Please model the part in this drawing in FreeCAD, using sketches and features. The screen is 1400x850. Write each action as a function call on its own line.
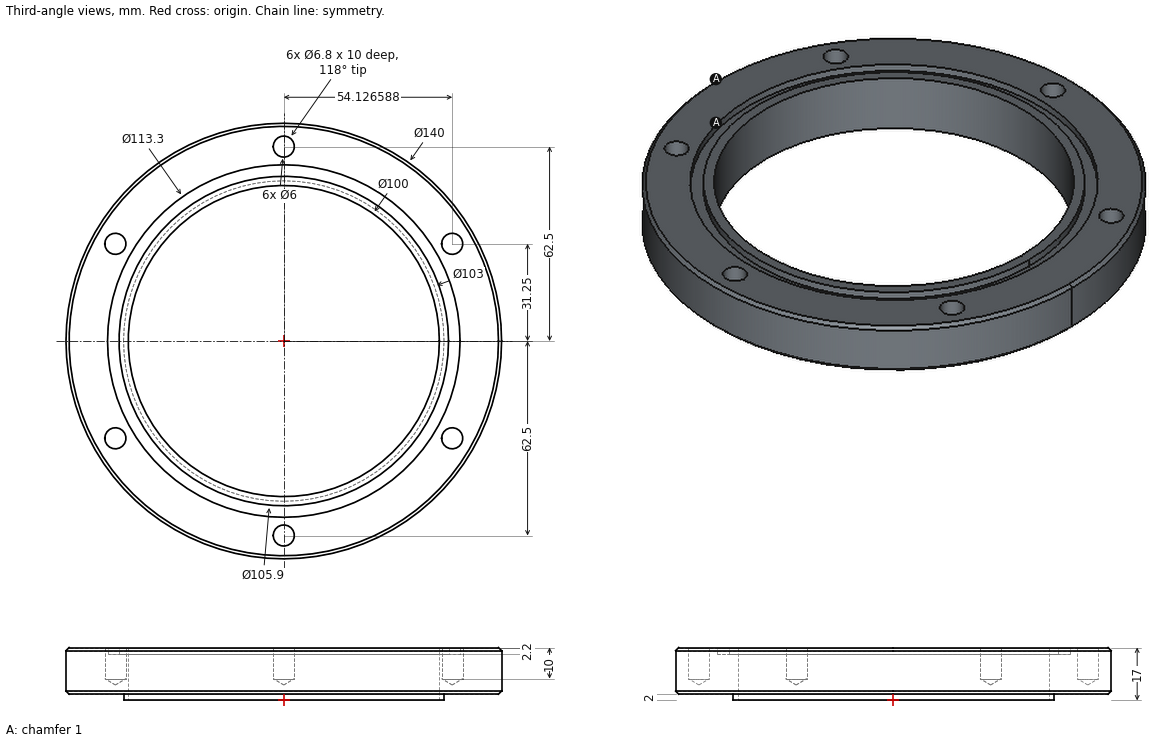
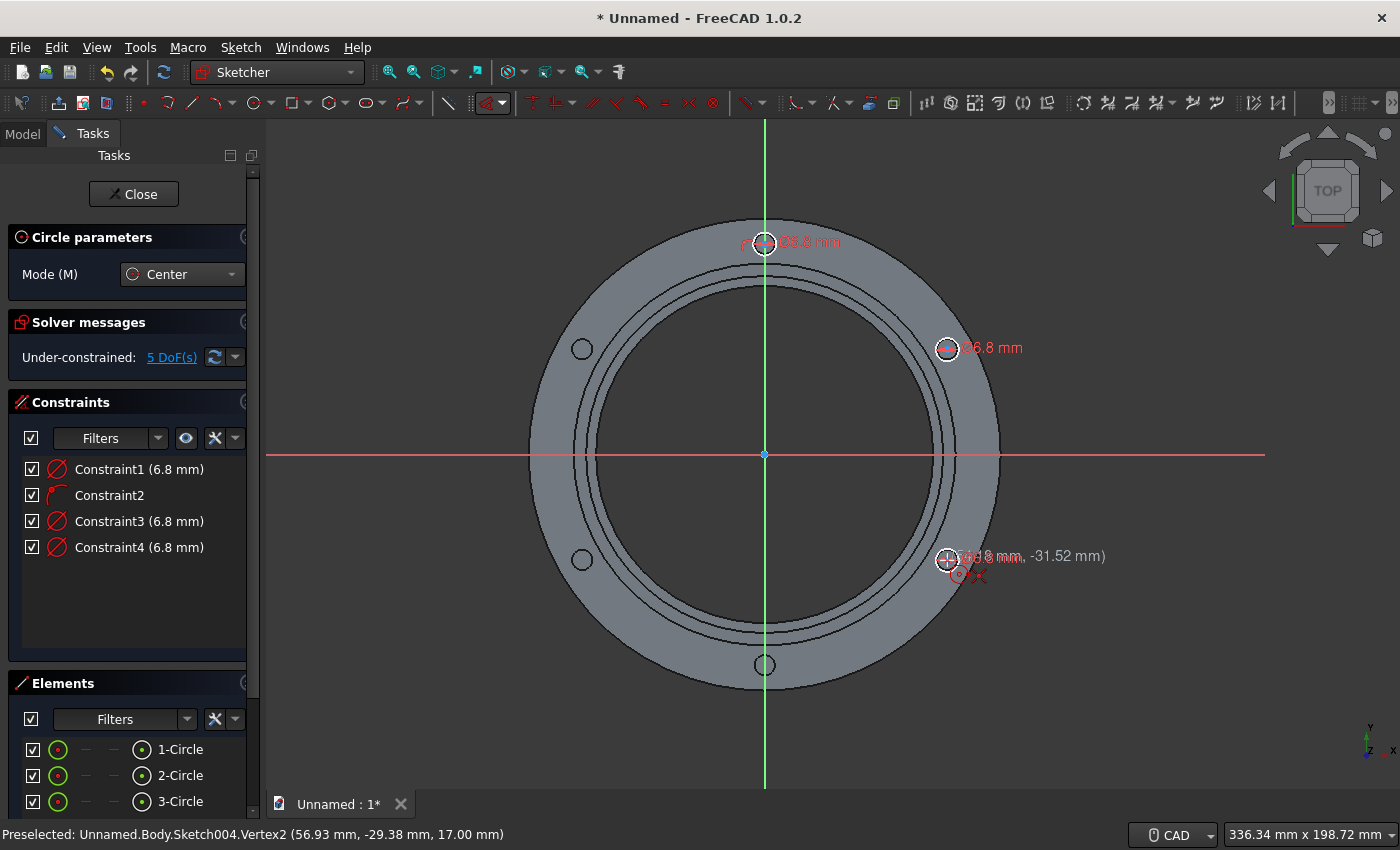
scroll(765, 665, up, 4)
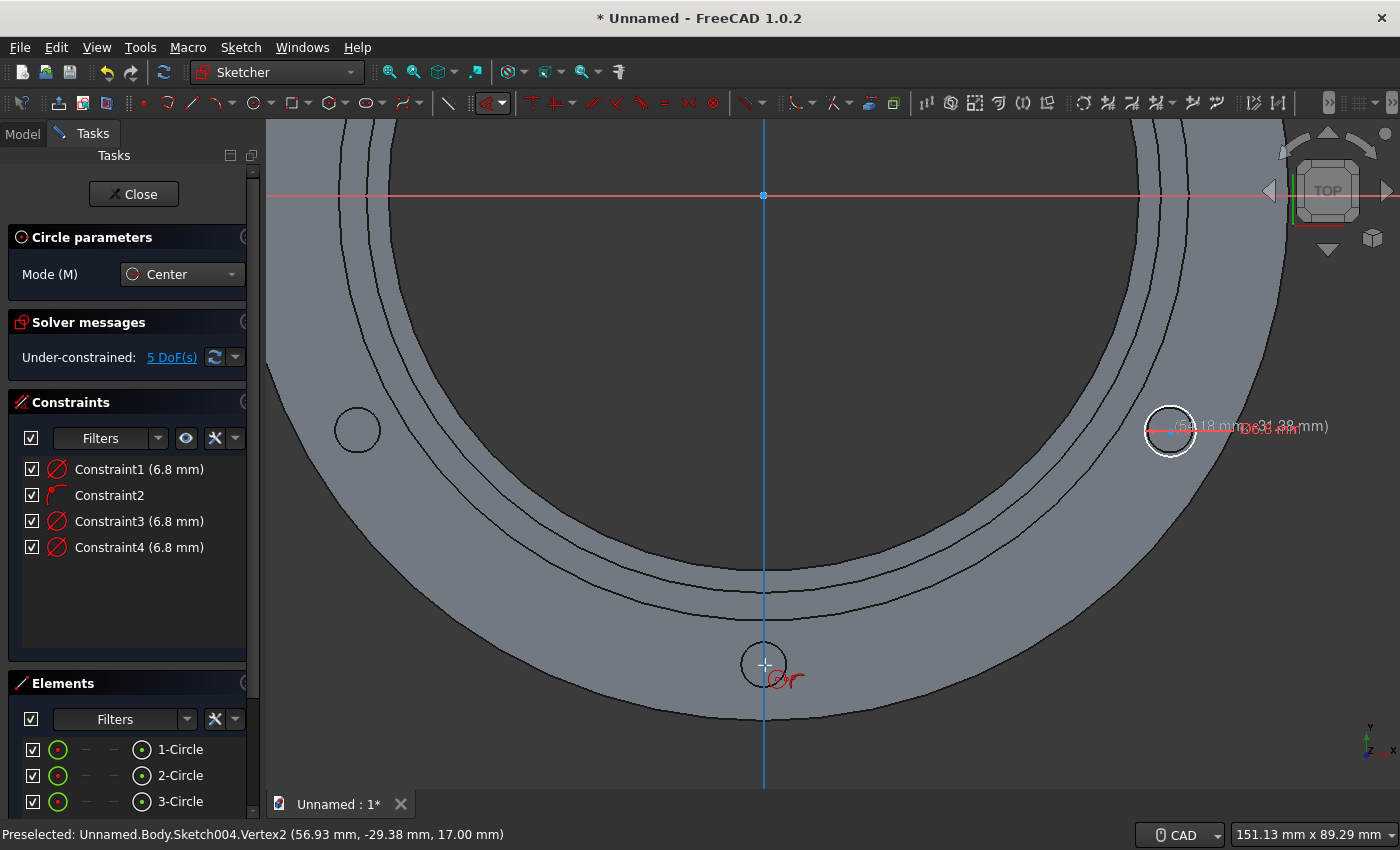
click(764, 665)
move(782, 647)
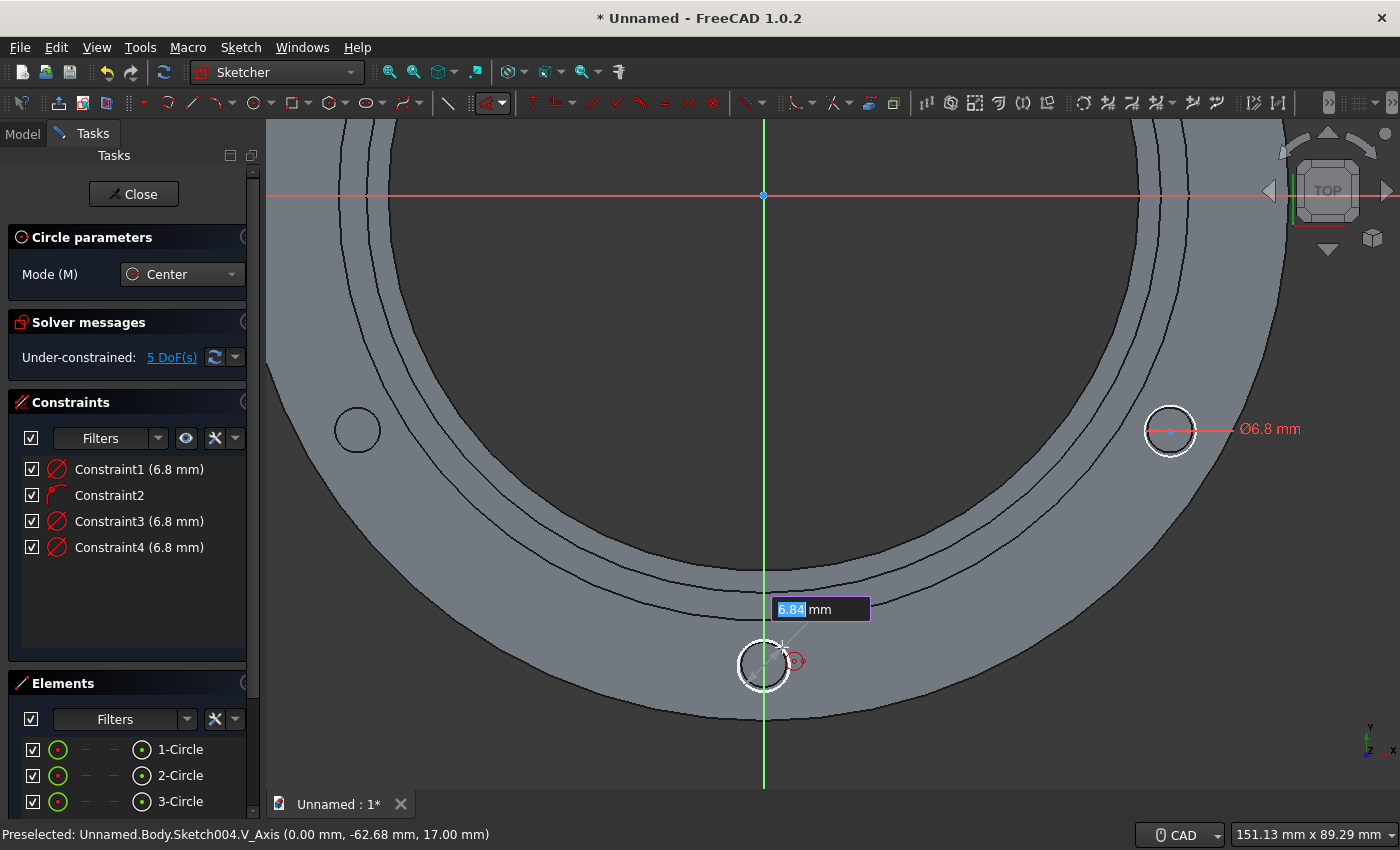
text(6.8)
key(Return)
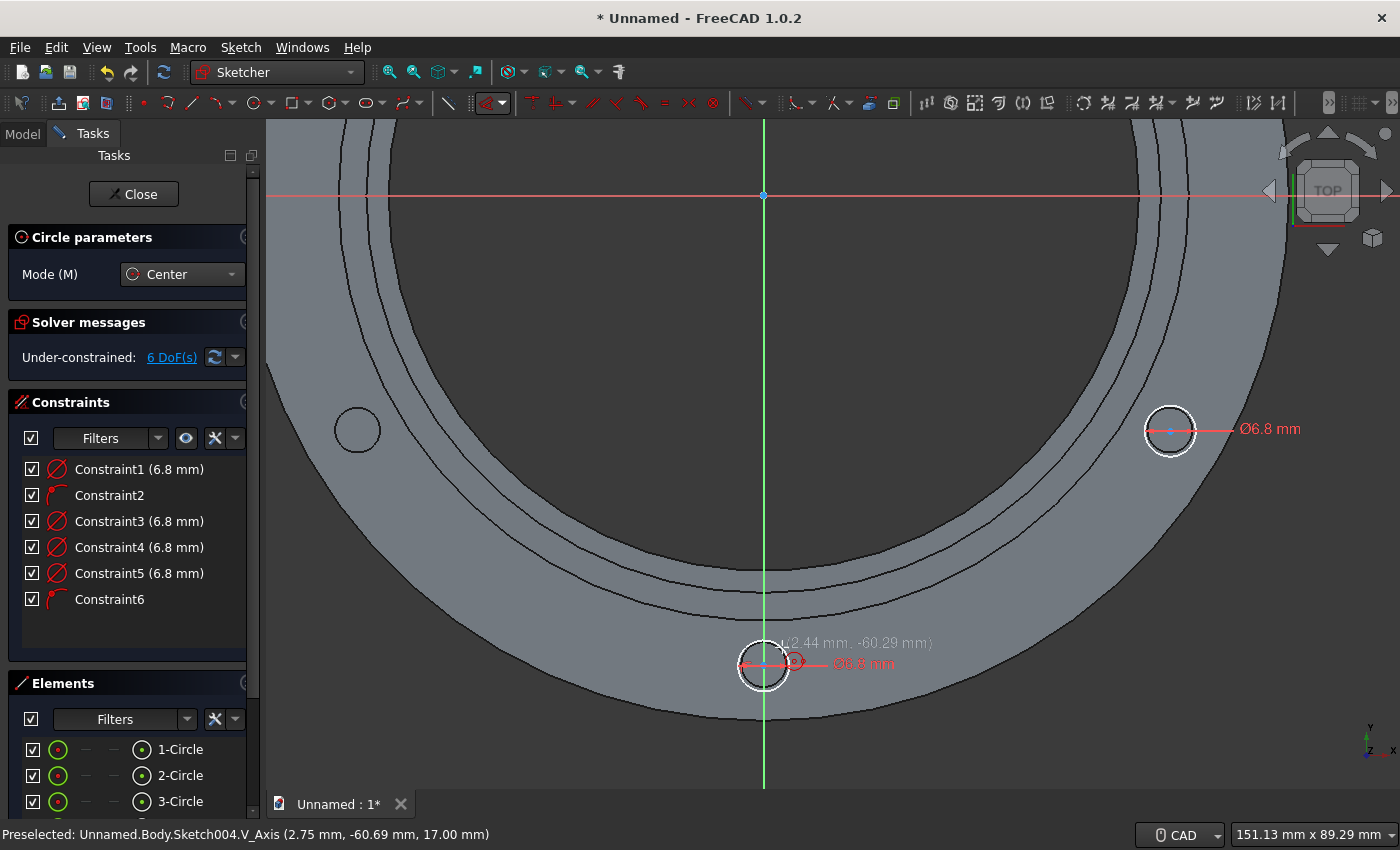
click(358, 430)
move(376, 412)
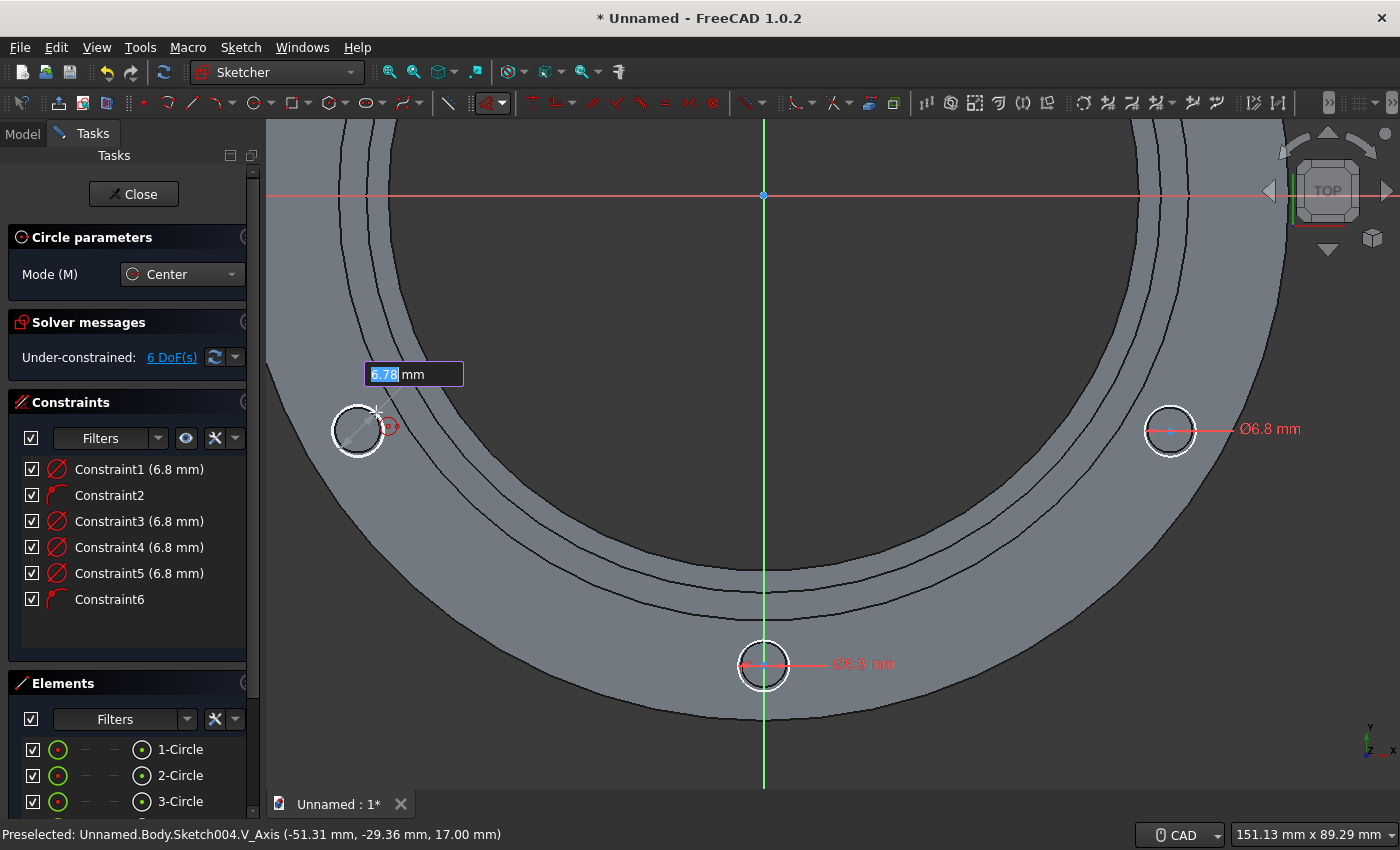
text(6.8)
key(Return)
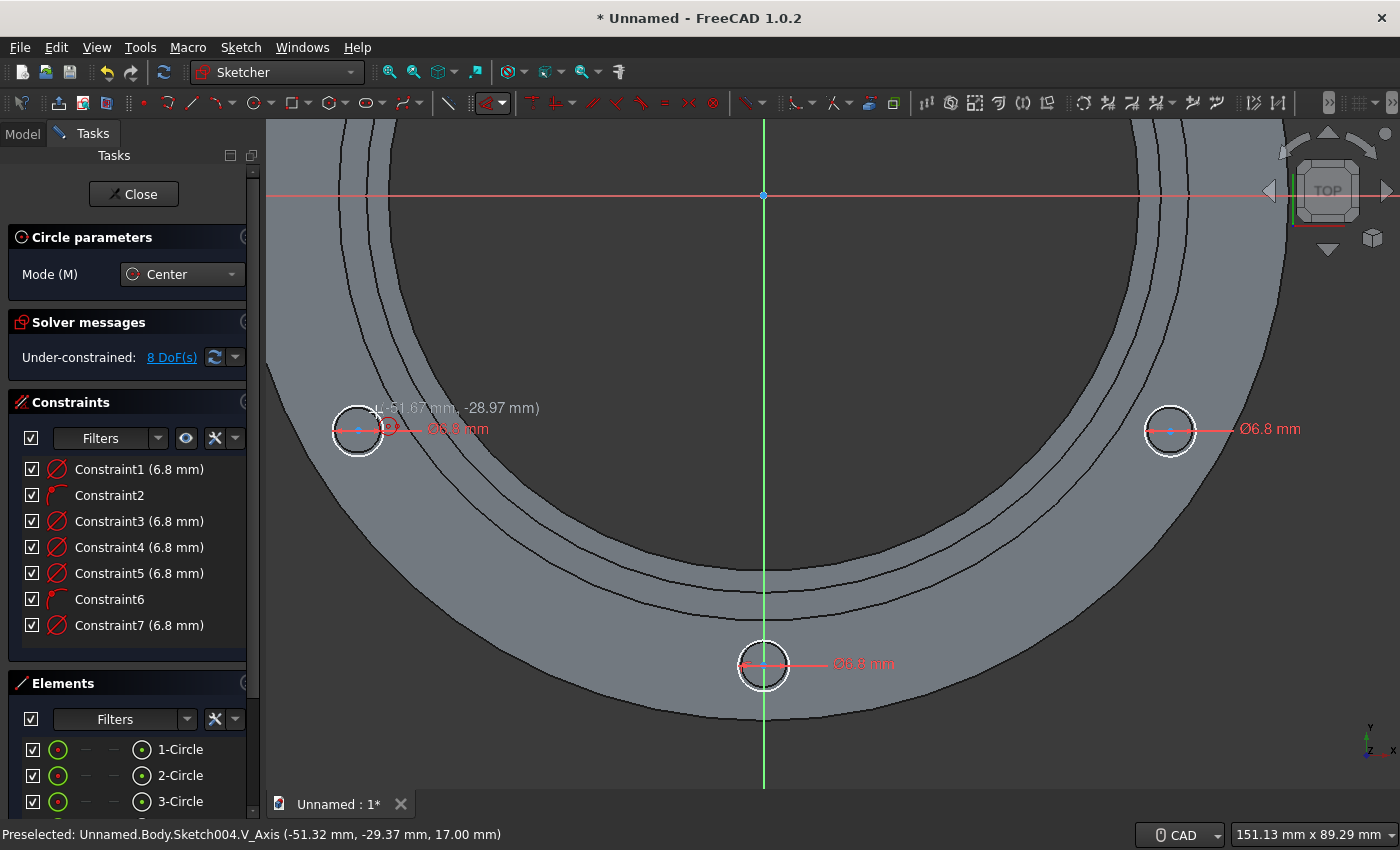
scroll(765, 665, down, 4)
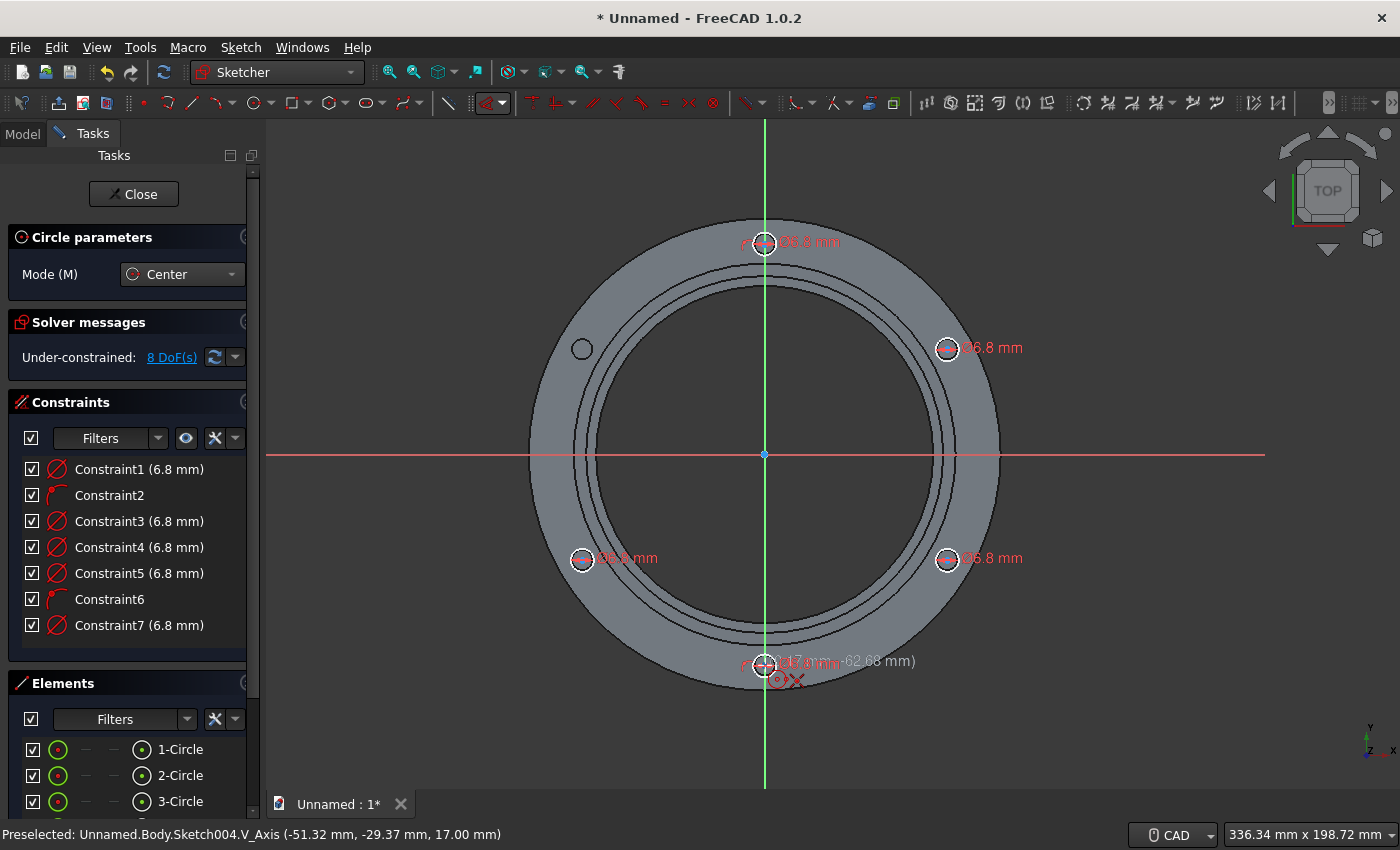
scroll(582, 349, up, 4)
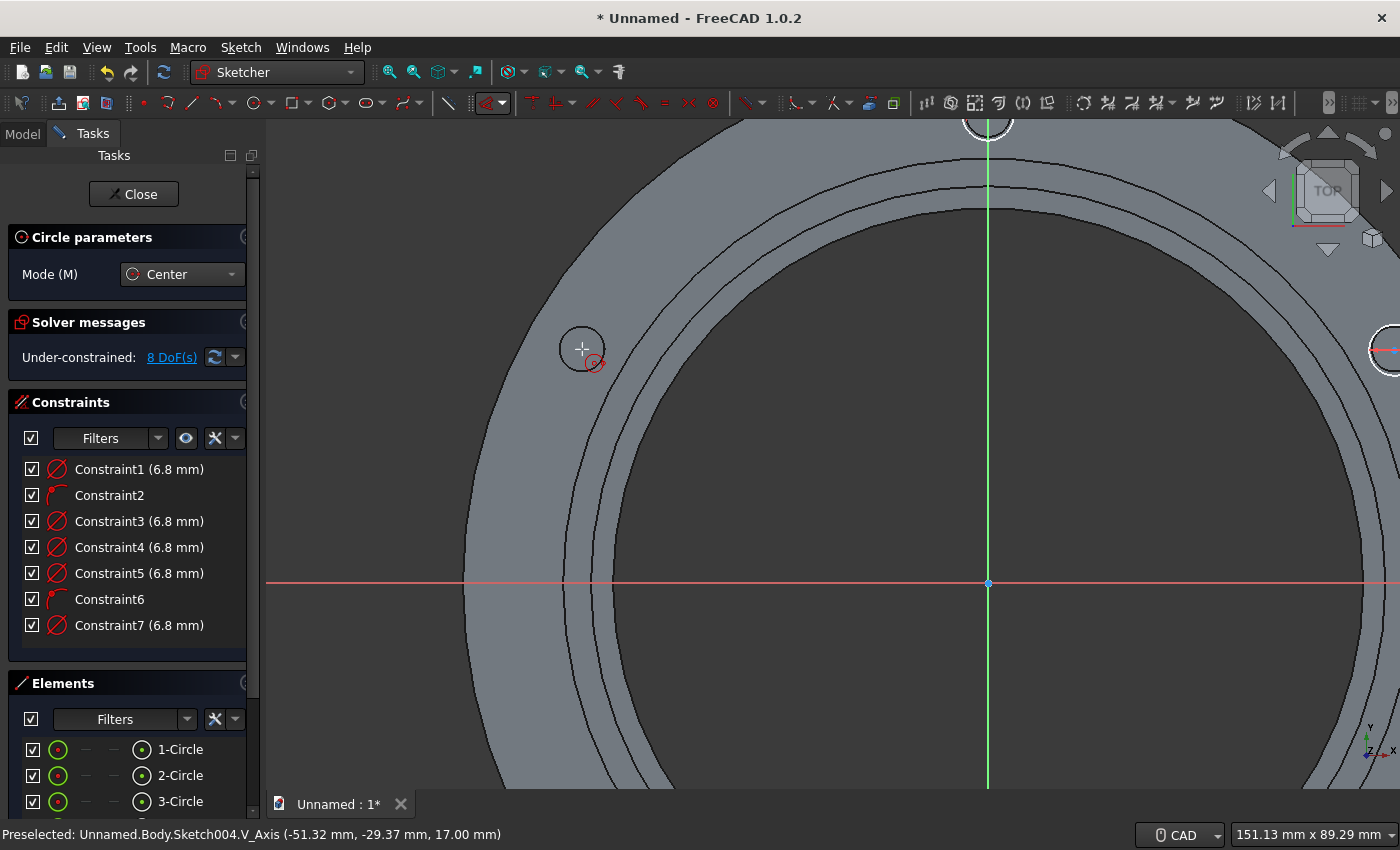
click(582, 349)
move(600, 331)